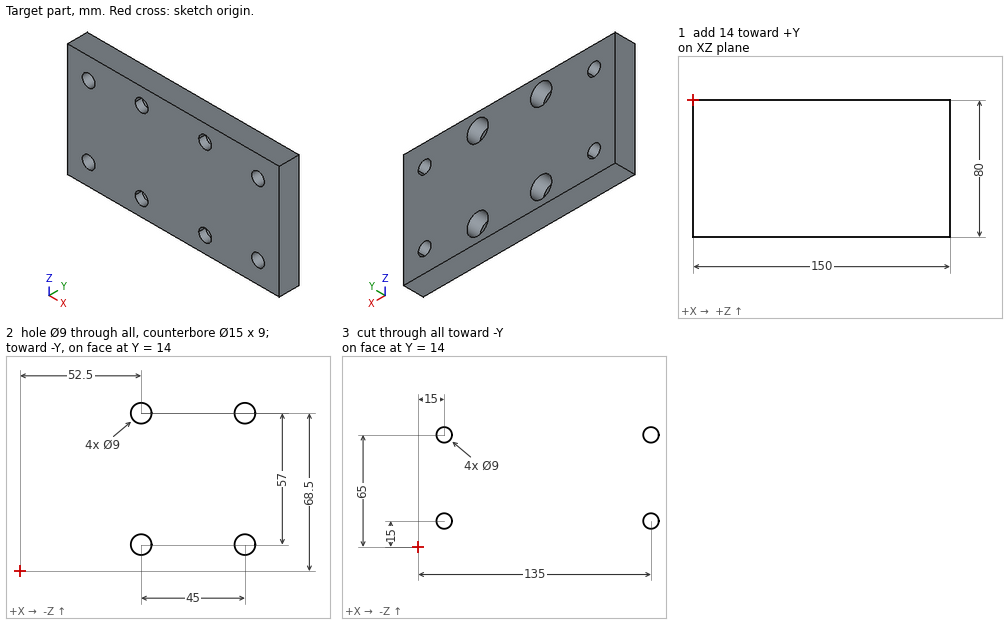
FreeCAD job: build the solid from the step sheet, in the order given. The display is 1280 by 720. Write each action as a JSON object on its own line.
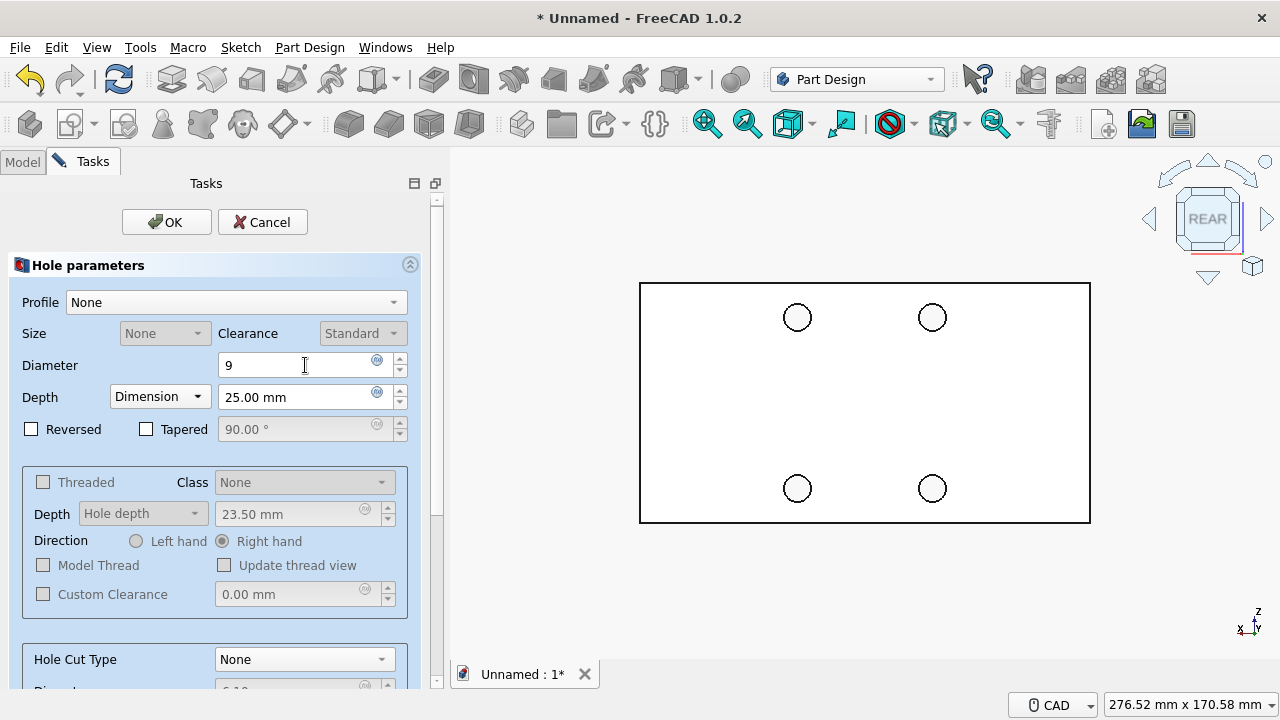
{"action": "left_click", "coordinate": [161, 396]}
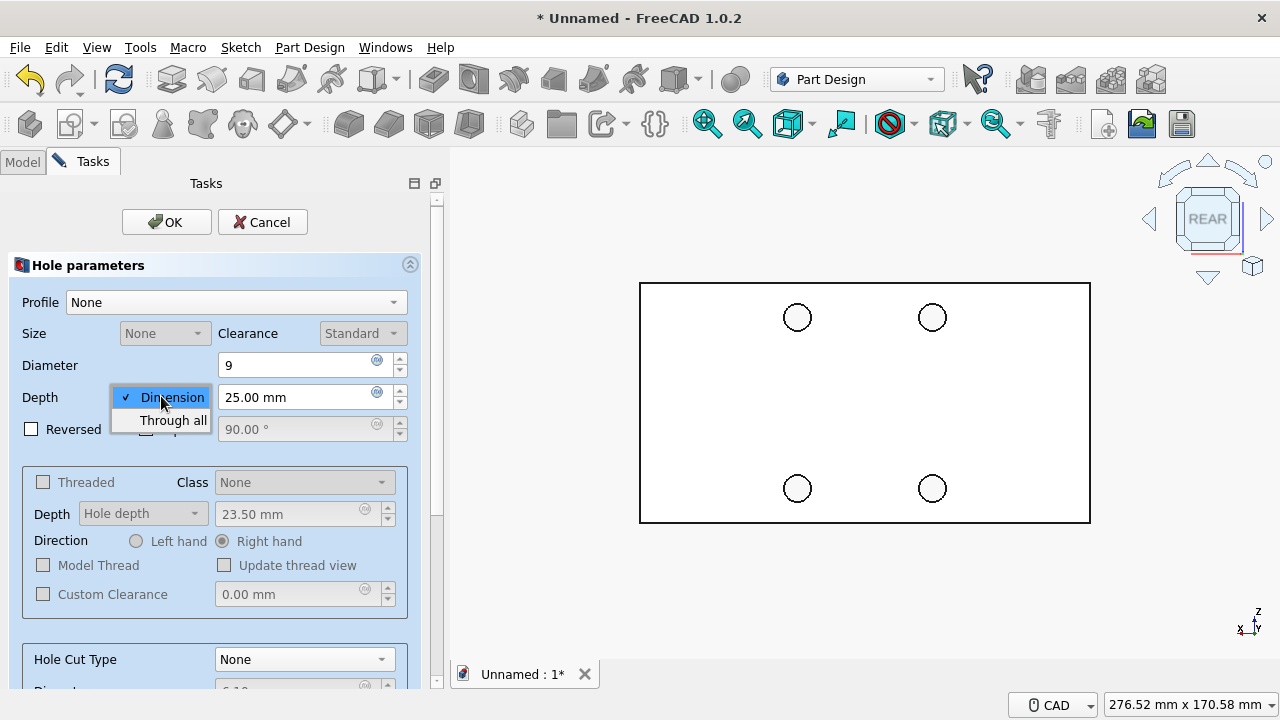
{"action": "left_click", "coordinate": [160, 420]}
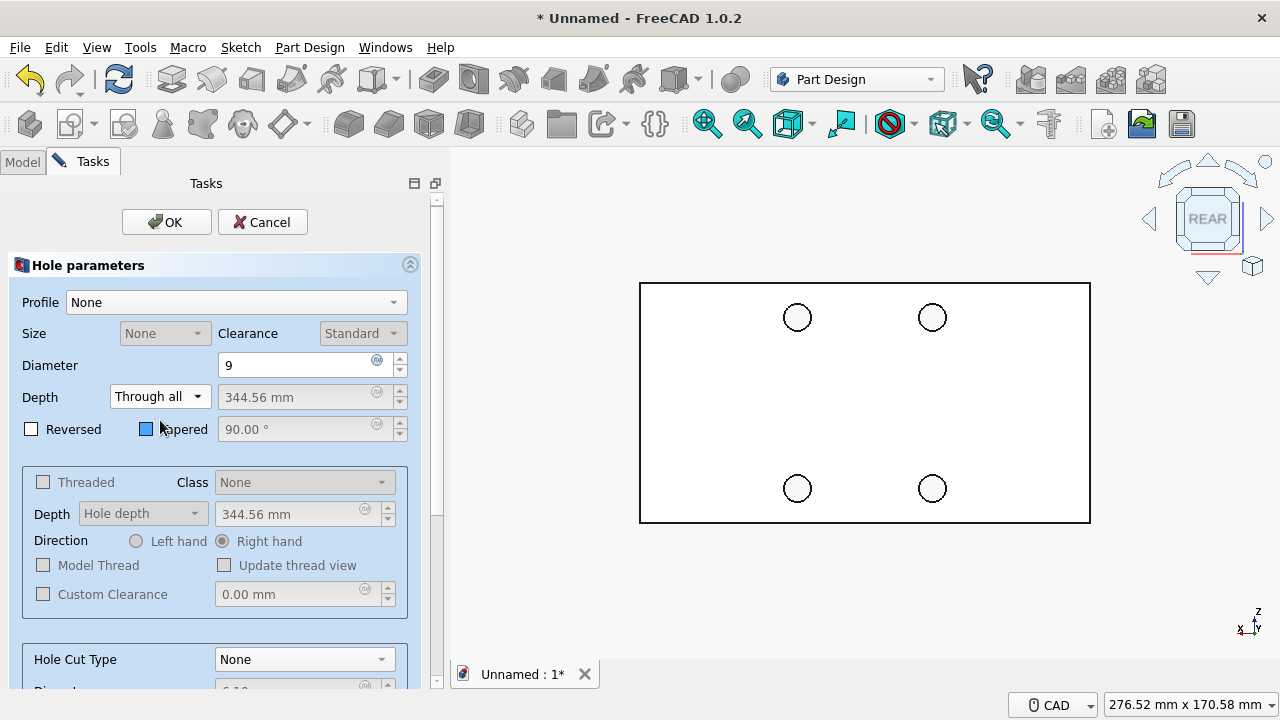
{"action": "left_click", "coordinate": [306, 660]}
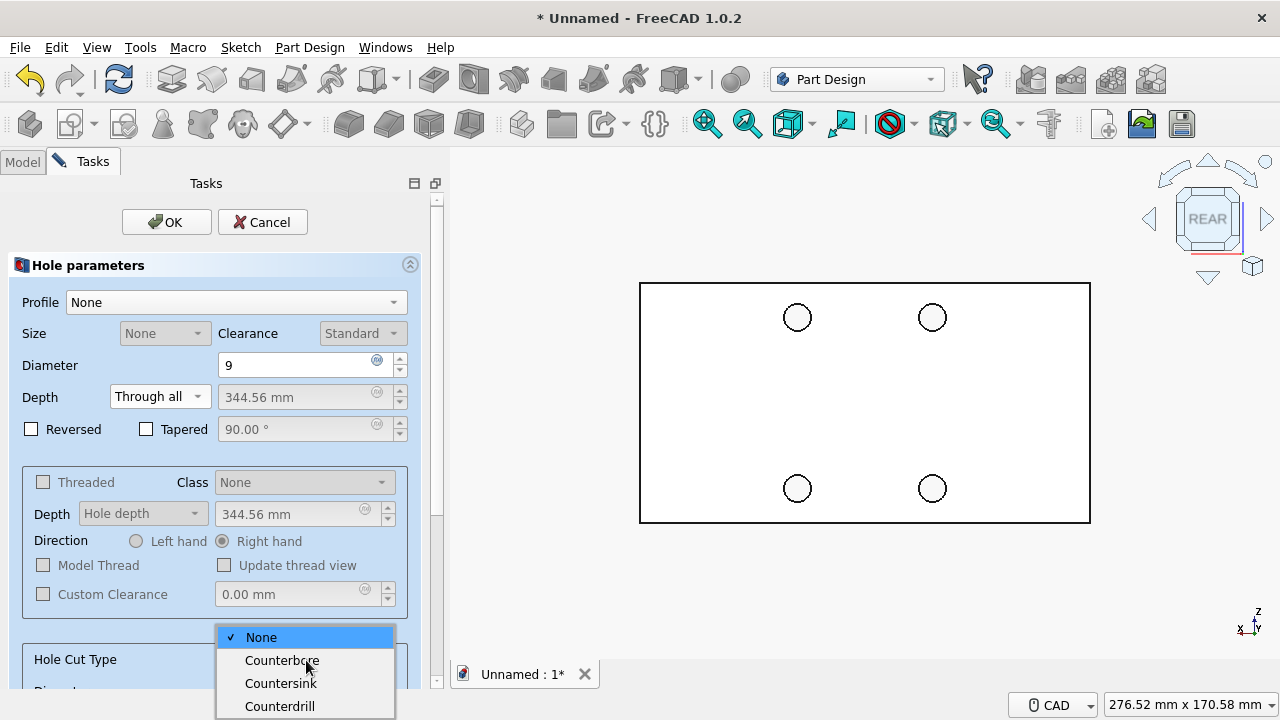
{"action": "left_click", "coordinate": [304, 660]}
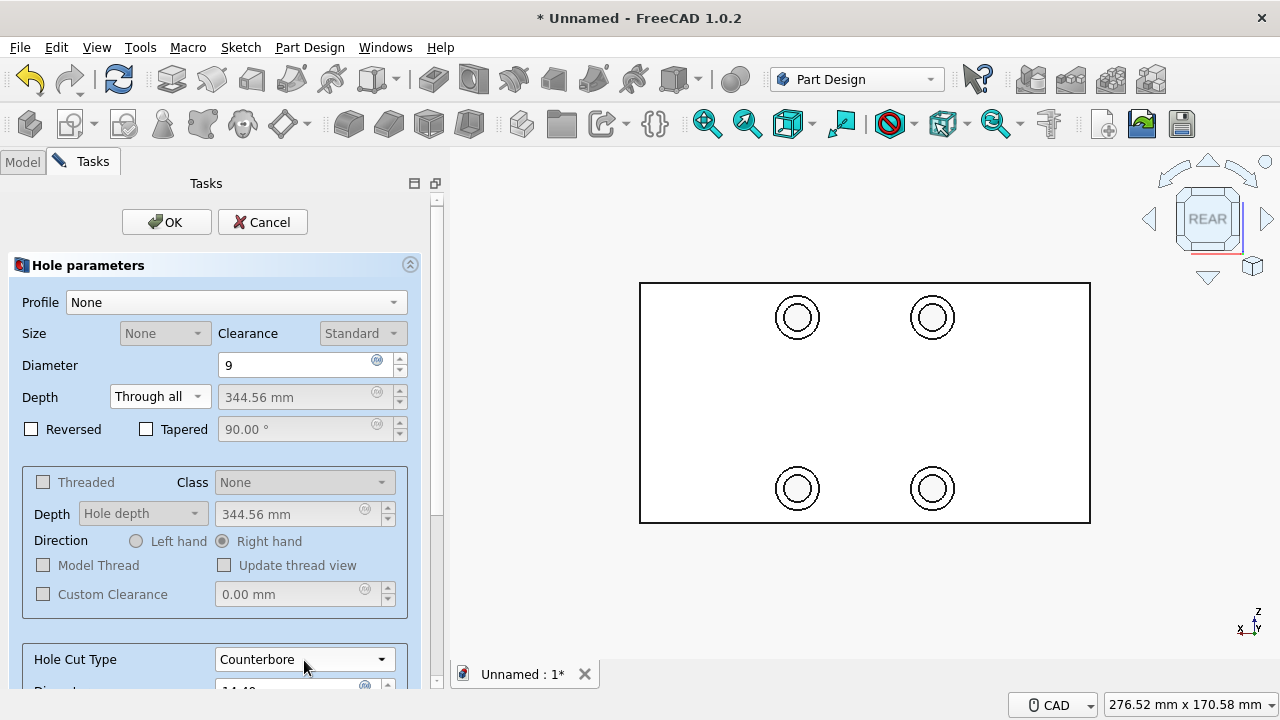
{"action": "scroll", "coordinate": [437, 440], "scroll_direction": "down", "scroll_amount": 2}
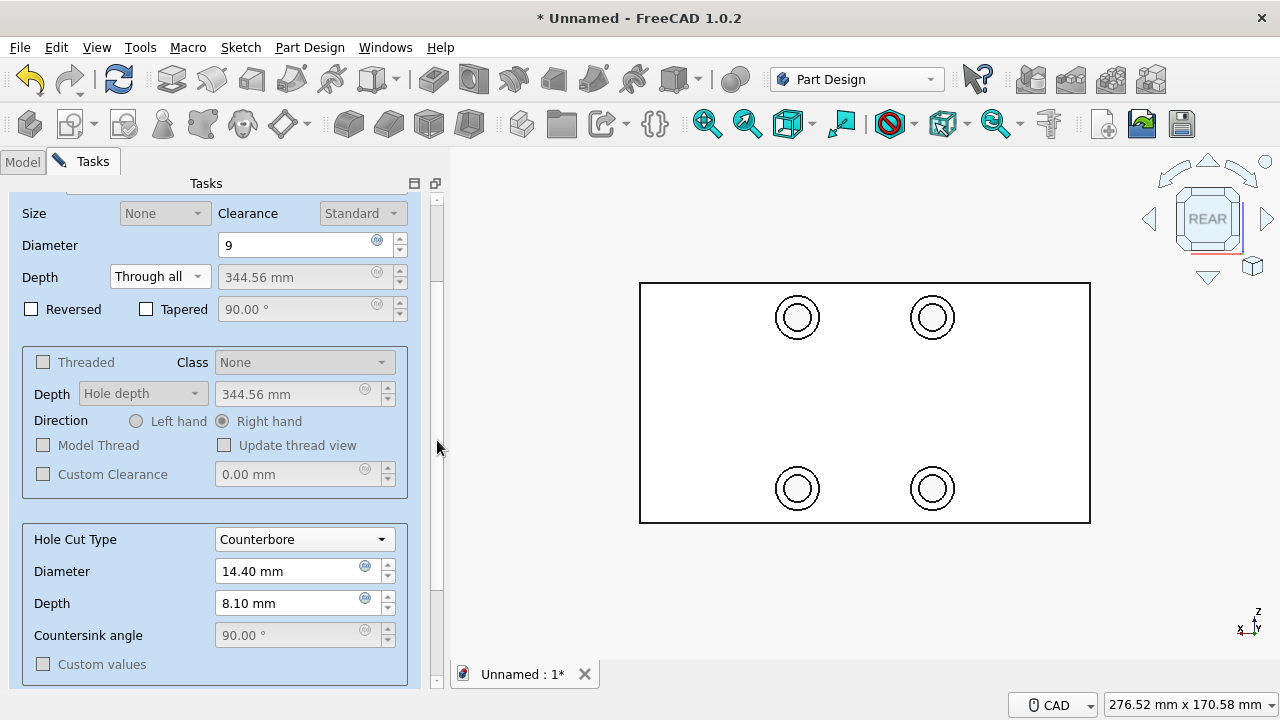
{"action": "triple_click", "coordinate": [298, 571]}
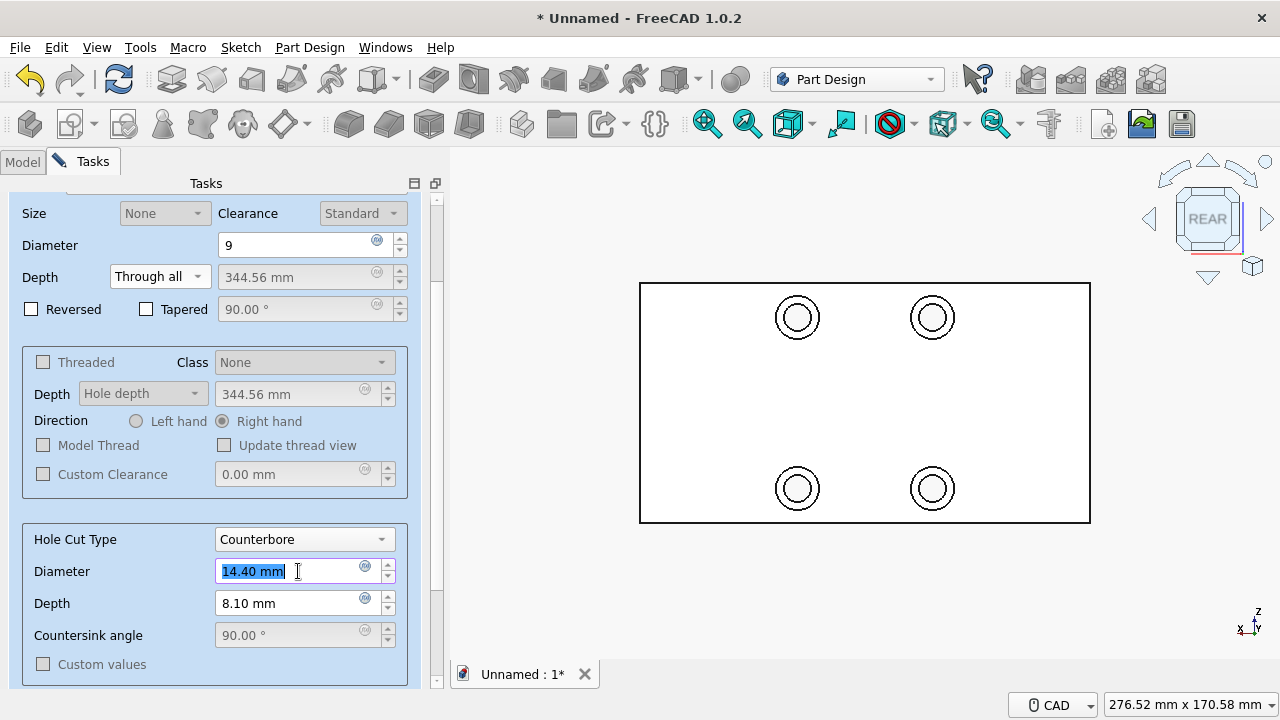
{"action": "type", "text": "15"}
{"action": "key", "text": "Tab"}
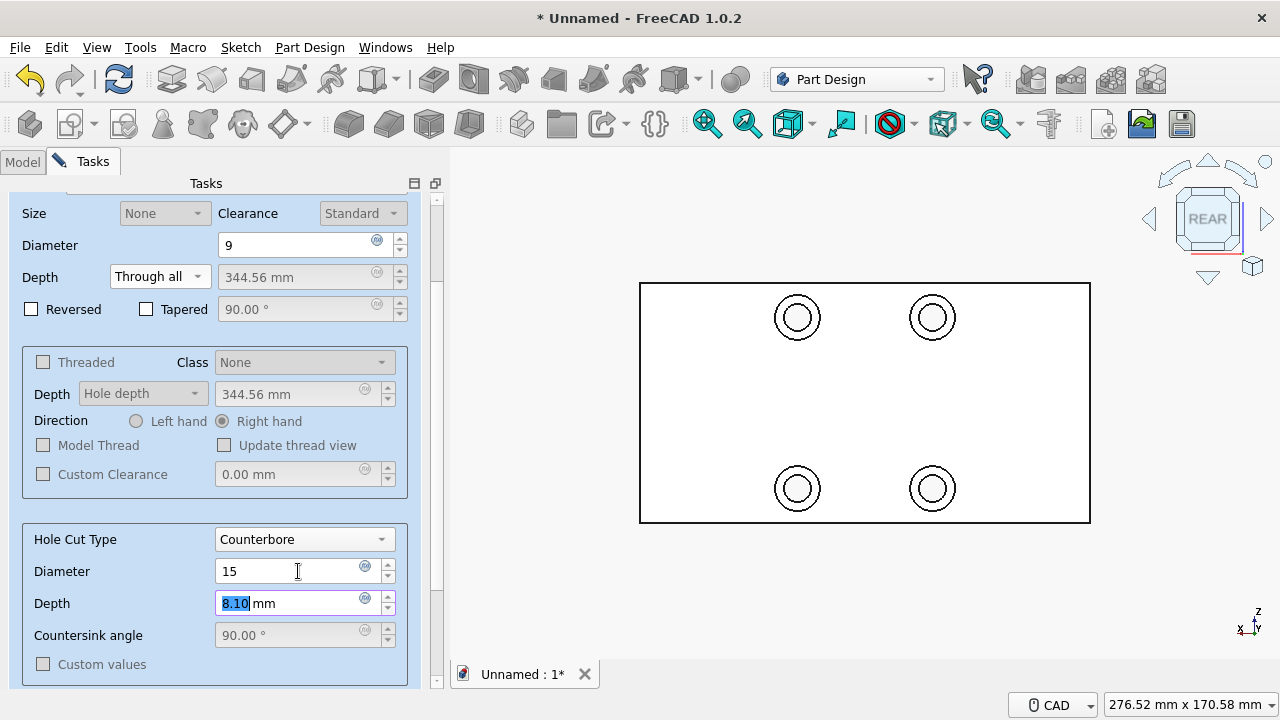
{"action": "type", "text": "9"}
{"action": "key", "text": "Tab"}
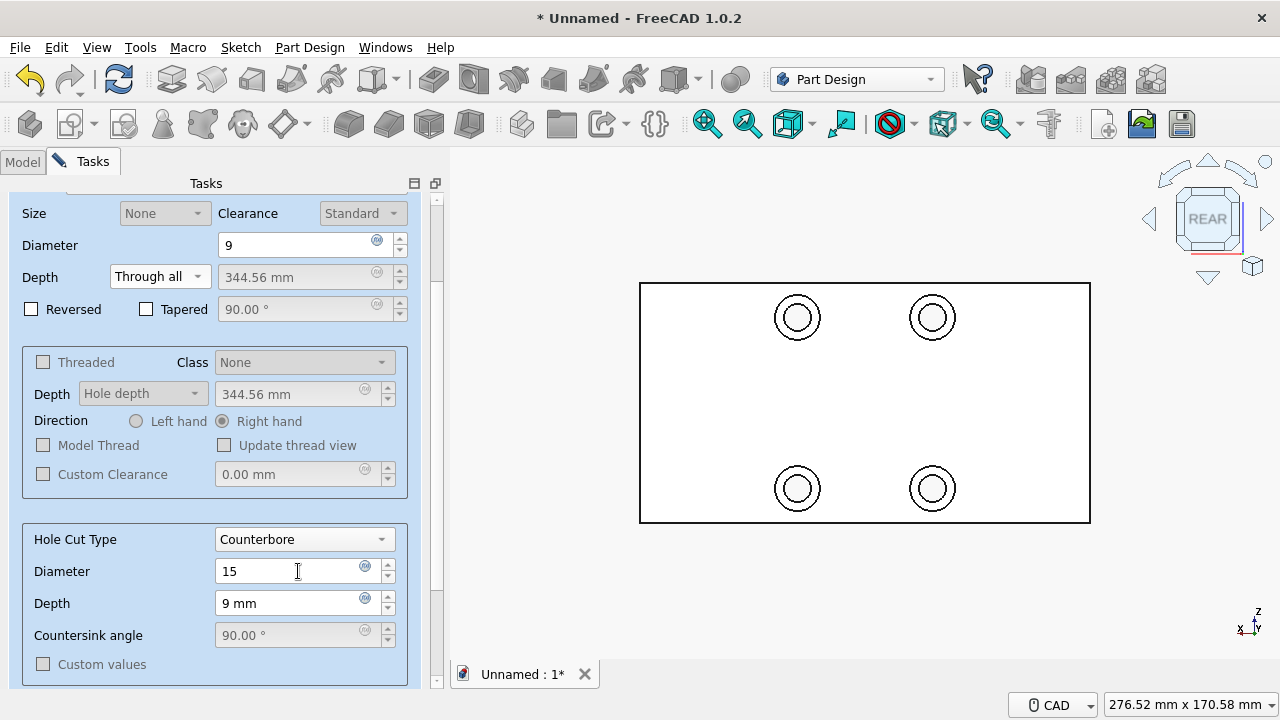
{"action": "scroll", "coordinate": [437, 440], "scroll_direction": "up", "scroll_amount": 3}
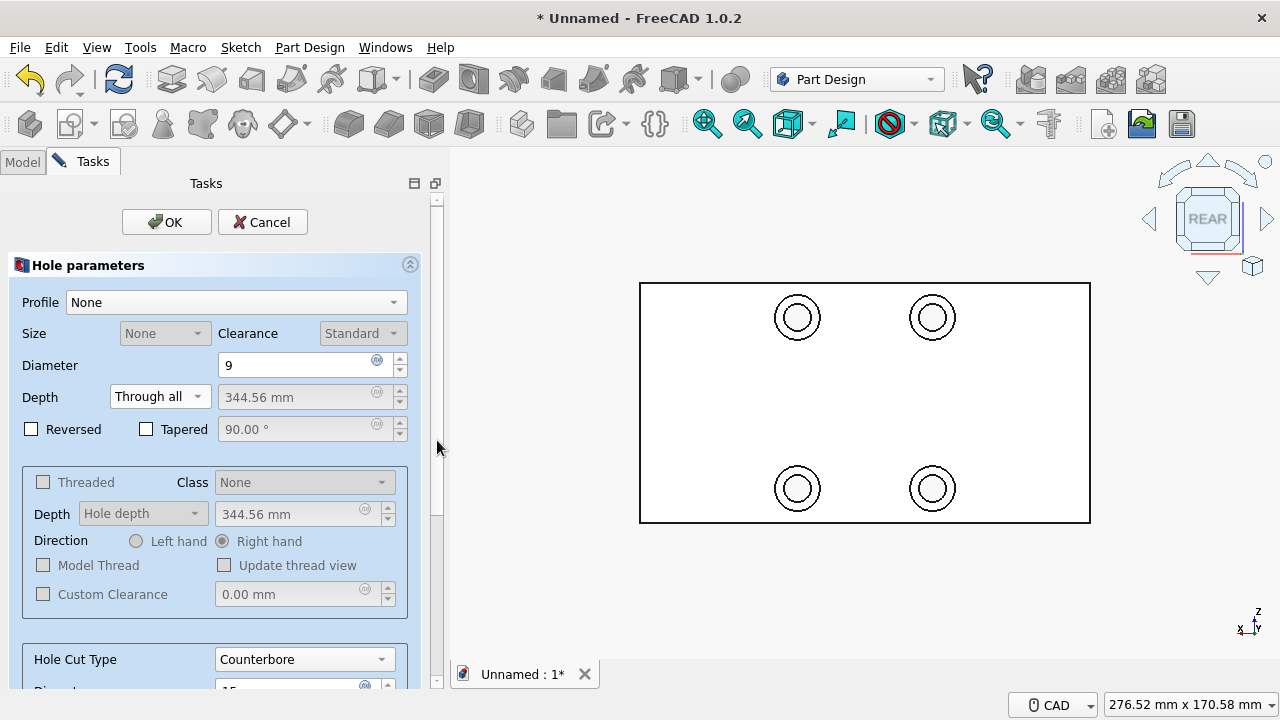
{"action": "left_click", "coordinate": [167, 222]}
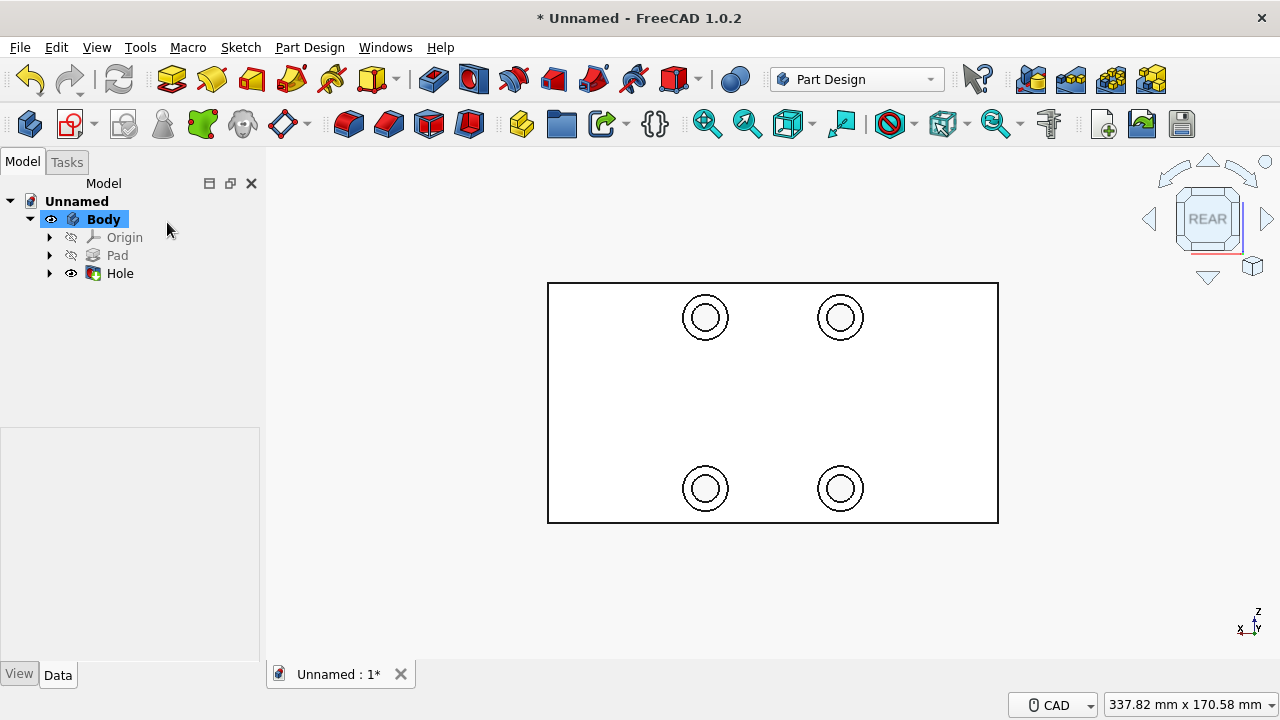
{"action": "left_click", "coordinate": [773, 402]}